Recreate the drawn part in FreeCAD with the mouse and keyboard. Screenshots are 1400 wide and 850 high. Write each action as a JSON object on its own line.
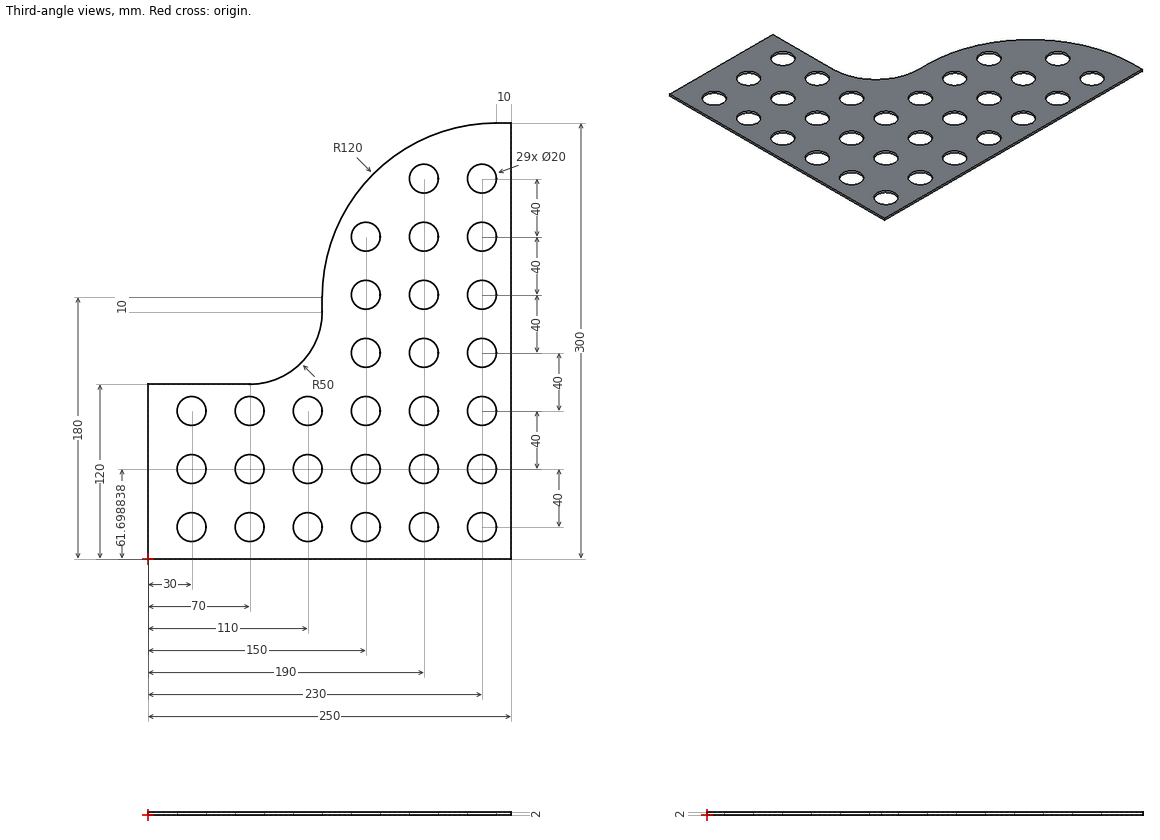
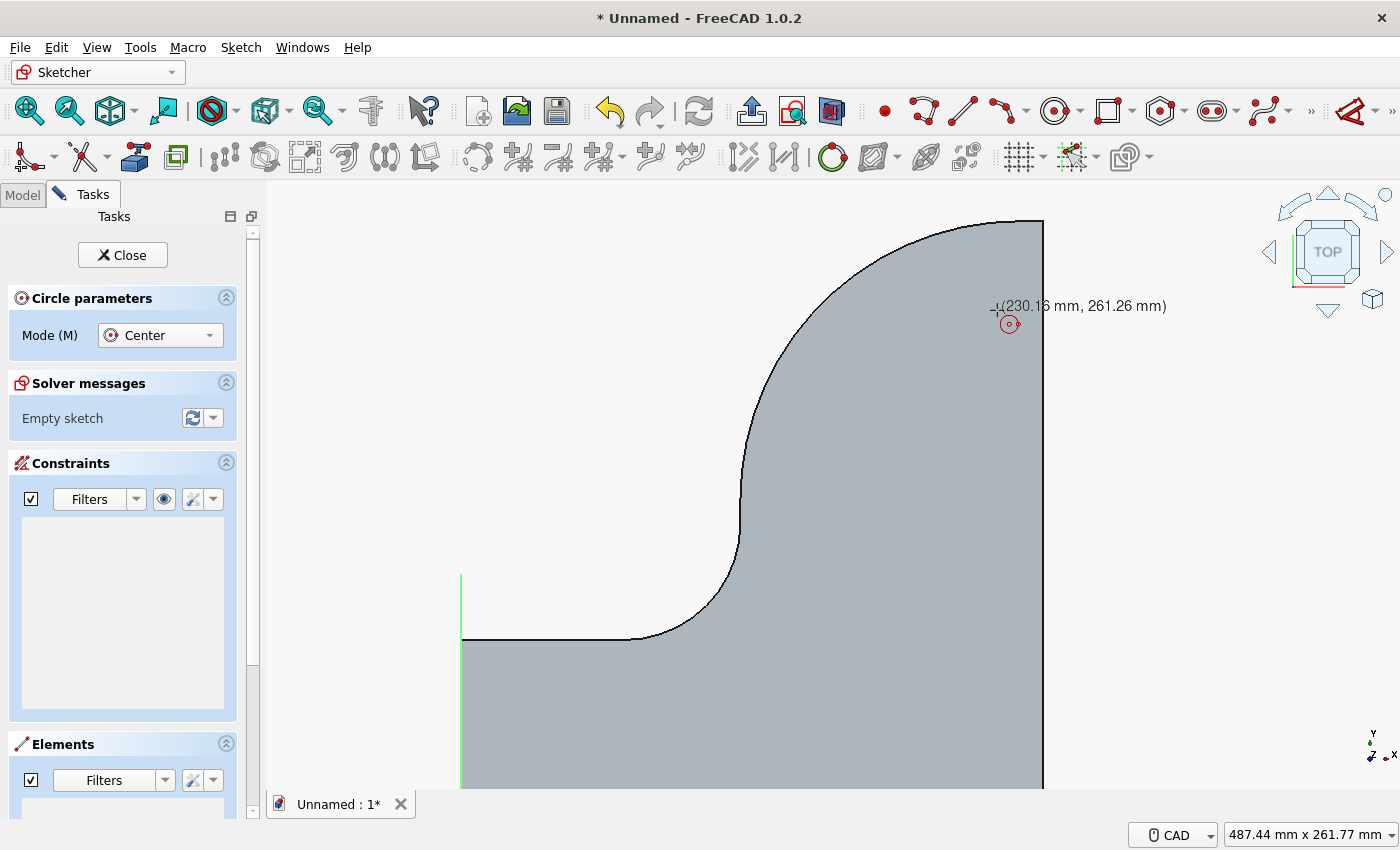
{"action": "left_click", "coordinate": [996, 310]}
{"action": "left_click", "coordinate": [1013, 294]}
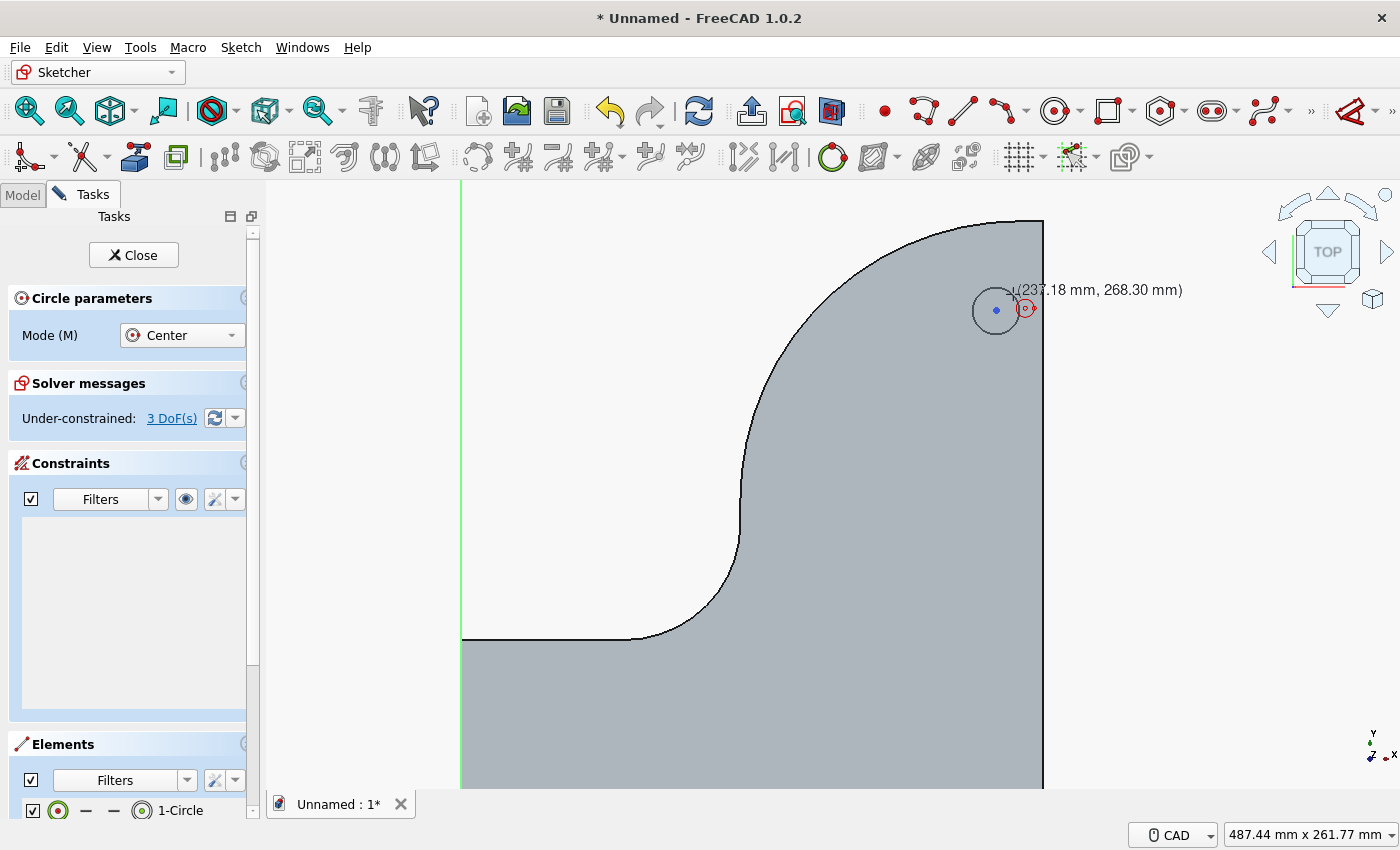
{"action": "left_click", "coordinate": [903, 310]}
{"action": "left_click", "coordinate": [920, 294]}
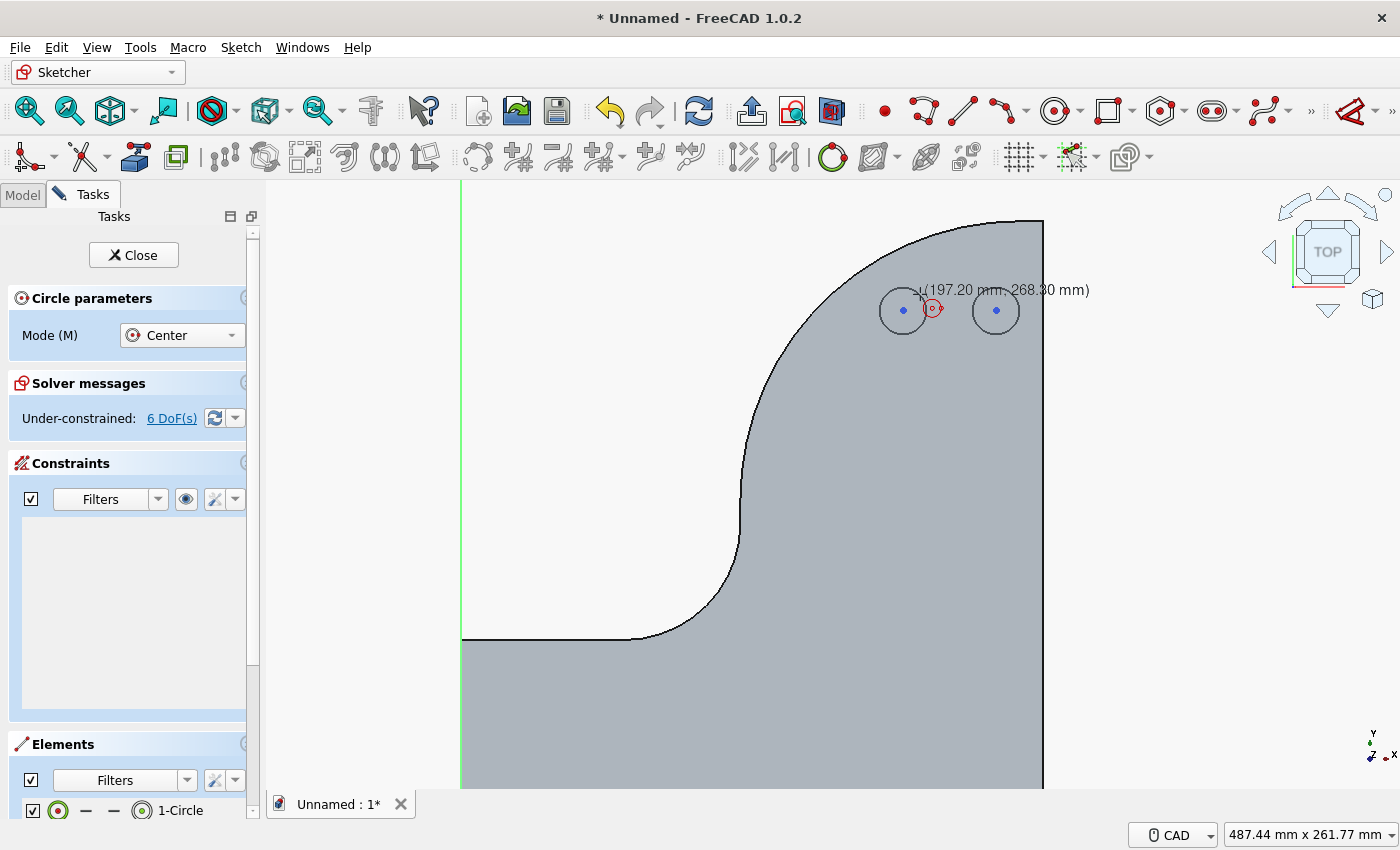
{"action": "left_click", "coordinate": [996, 403]}
{"action": "left_click", "coordinate": [1013, 387]}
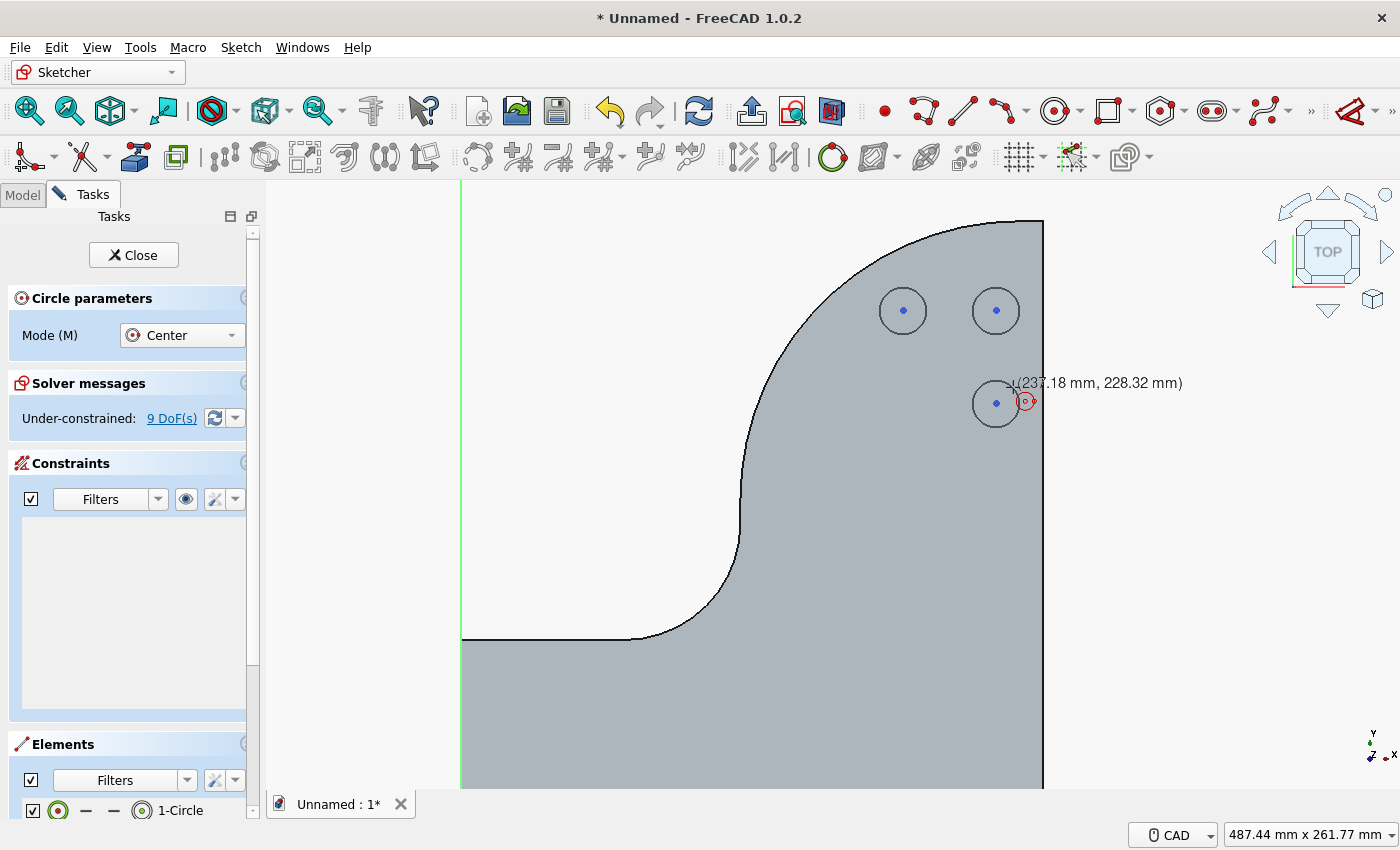
{"action": "left_click", "coordinate": [903, 403]}
{"action": "left_click", "coordinate": [920, 387]}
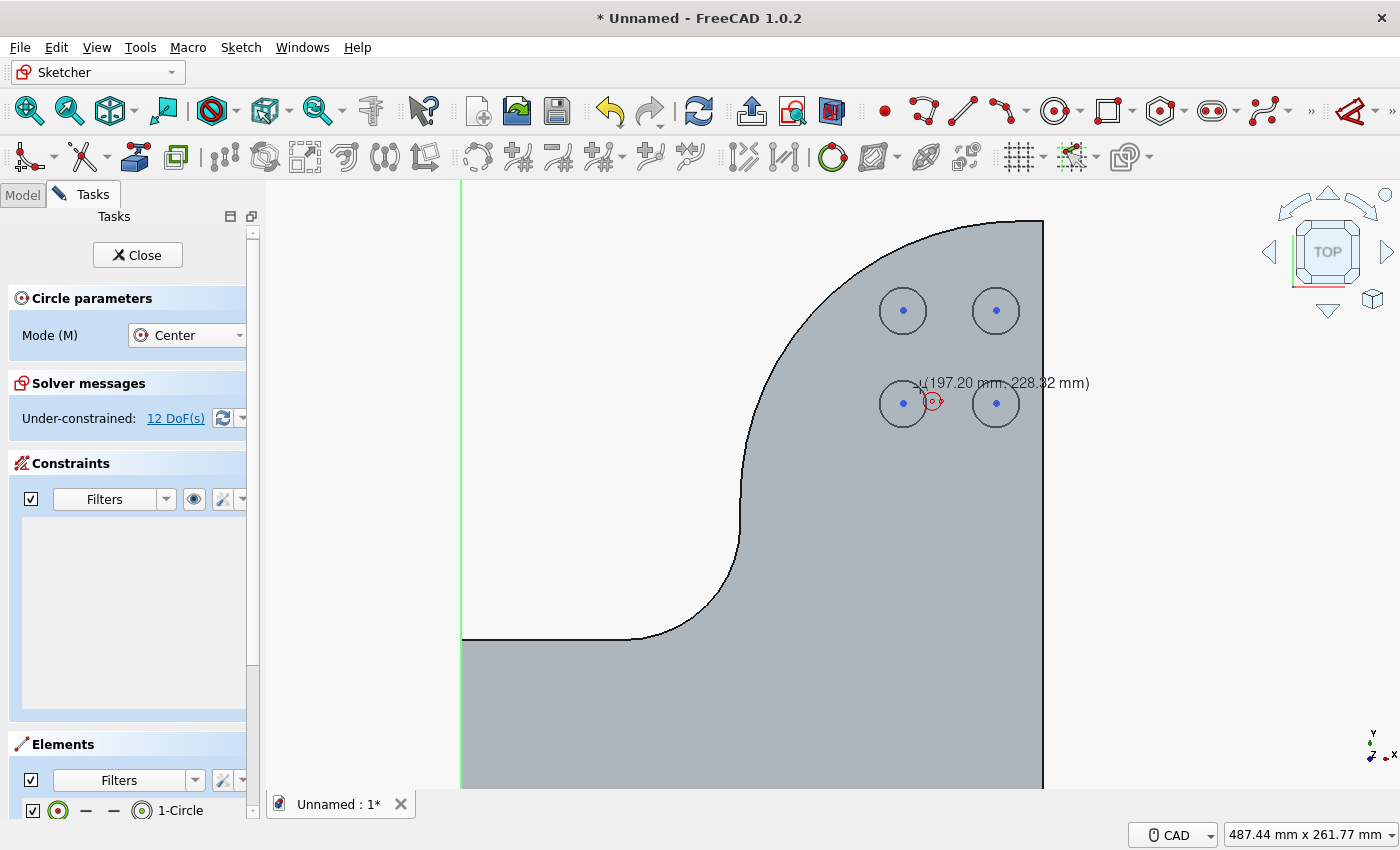
{"action": "left_click", "coordinate": [996, 496]}
{"action": "left_click", "coordinate": [1013, 480]}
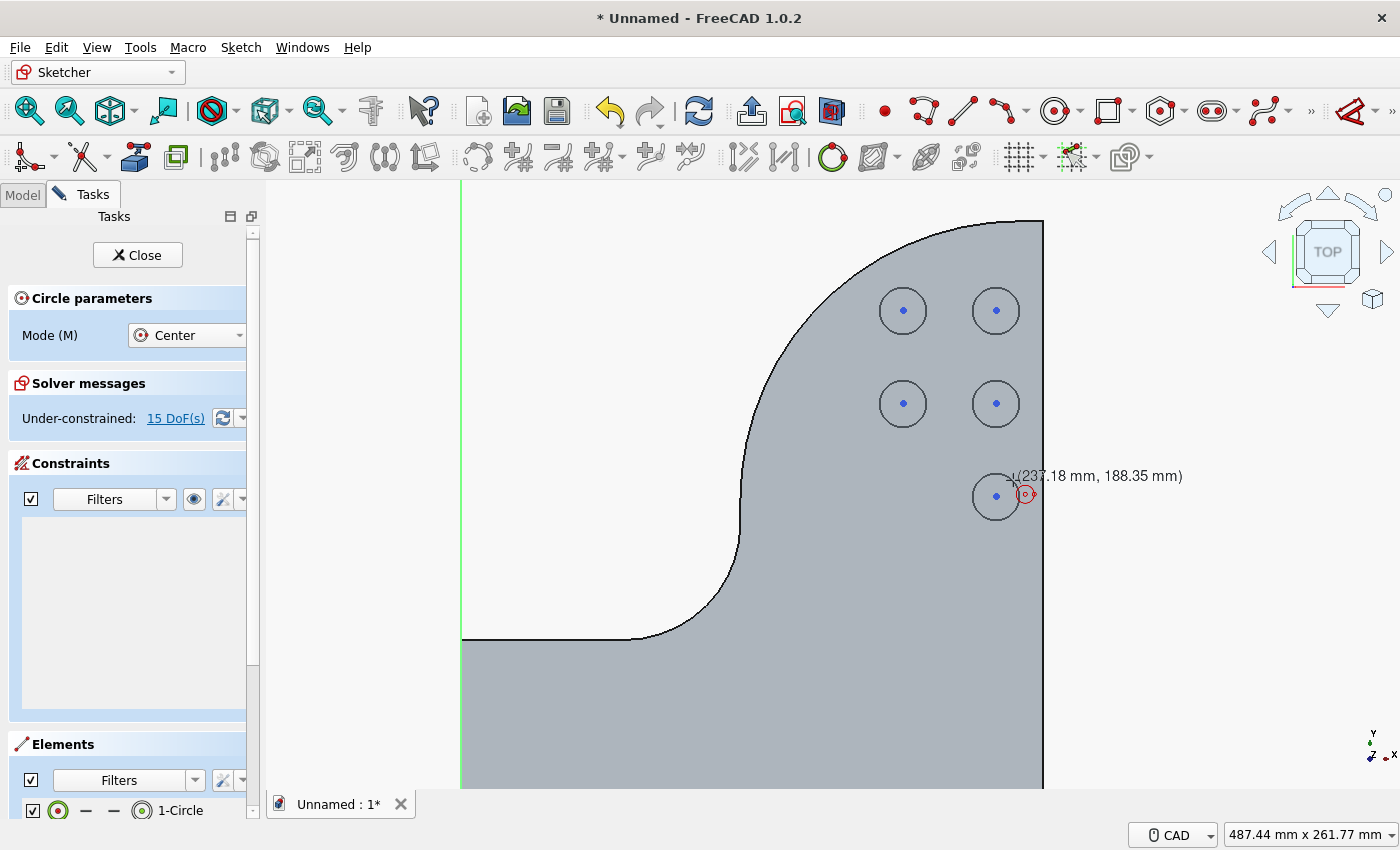
{"action": "left_click", "coordinate": [903, 496]}
{"action": "left_click", "coordinate": [920, 480]}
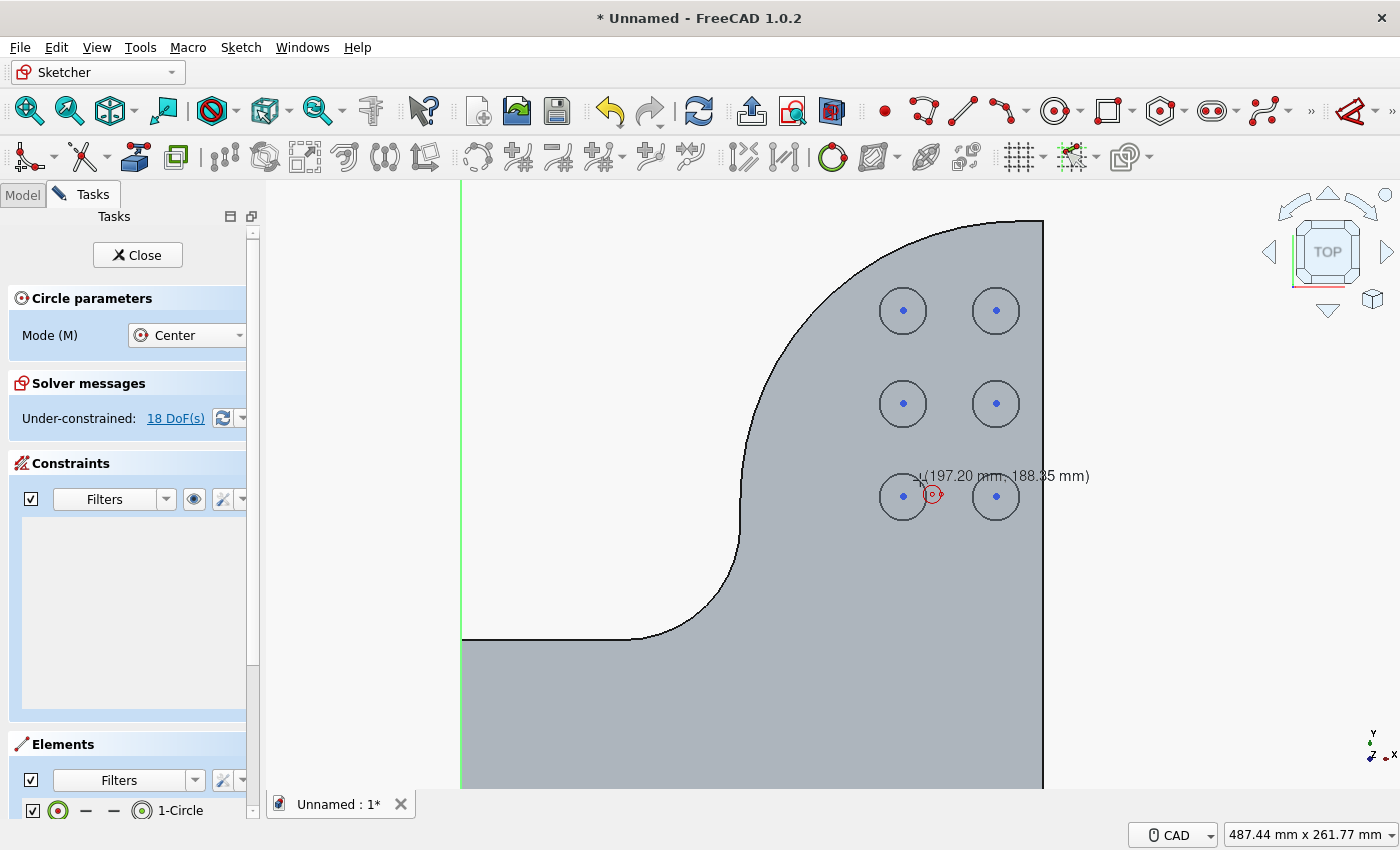
{"action": "left_click", "coordinate": [996, 590]}
{"action": "left_click", "coordinate": [1013, 573]}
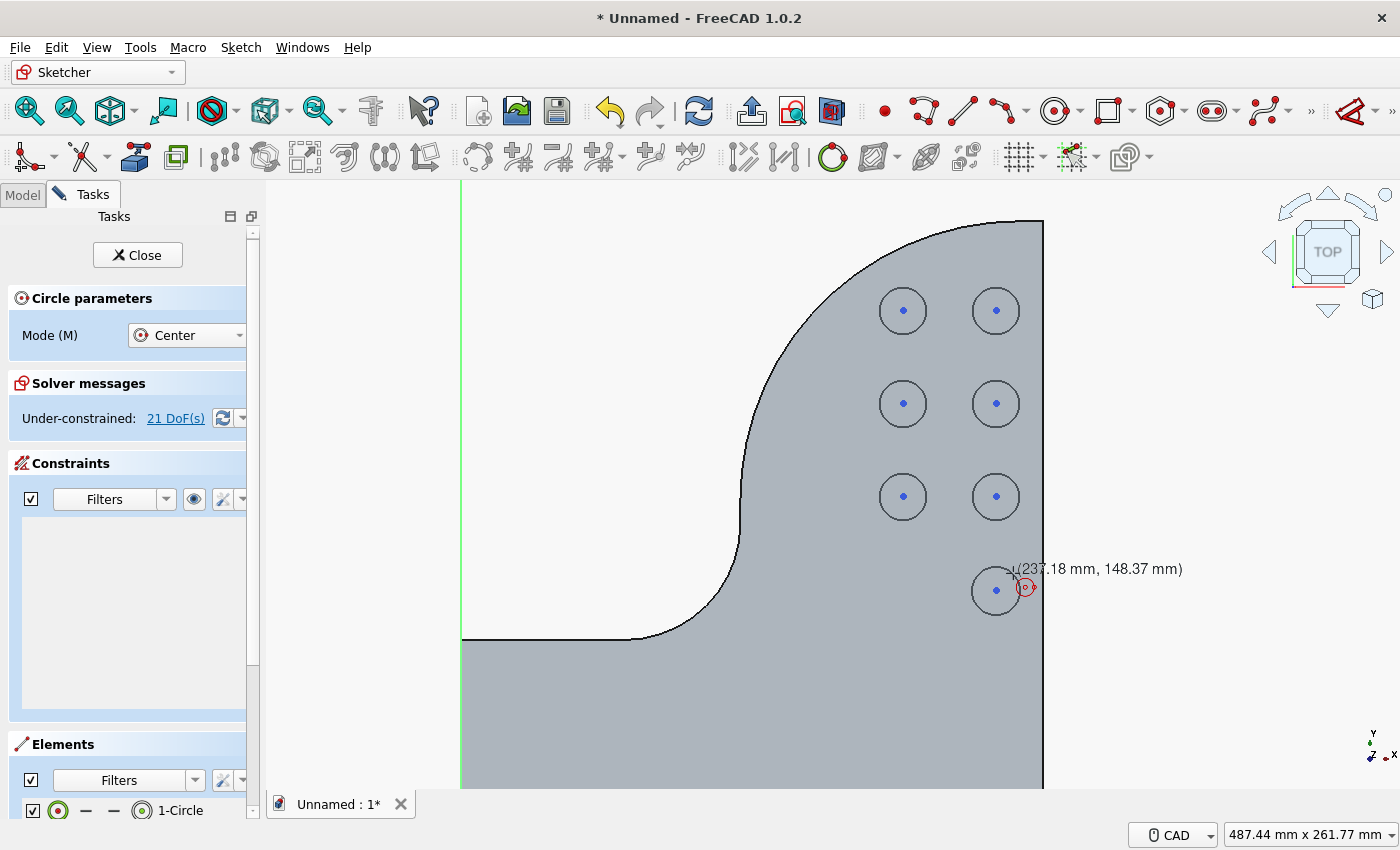
{"action": "left_click", "coordinate": [903, 590]}
{"action": "left_click", "coordinate": [920, 573]}